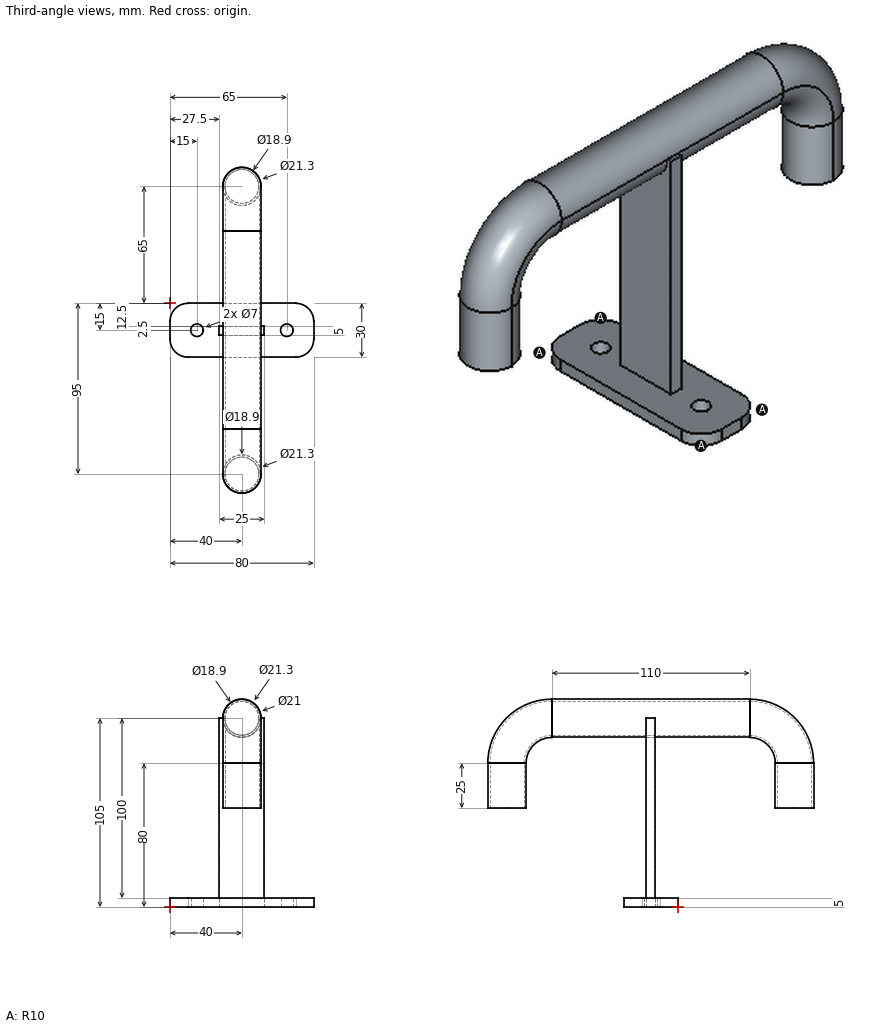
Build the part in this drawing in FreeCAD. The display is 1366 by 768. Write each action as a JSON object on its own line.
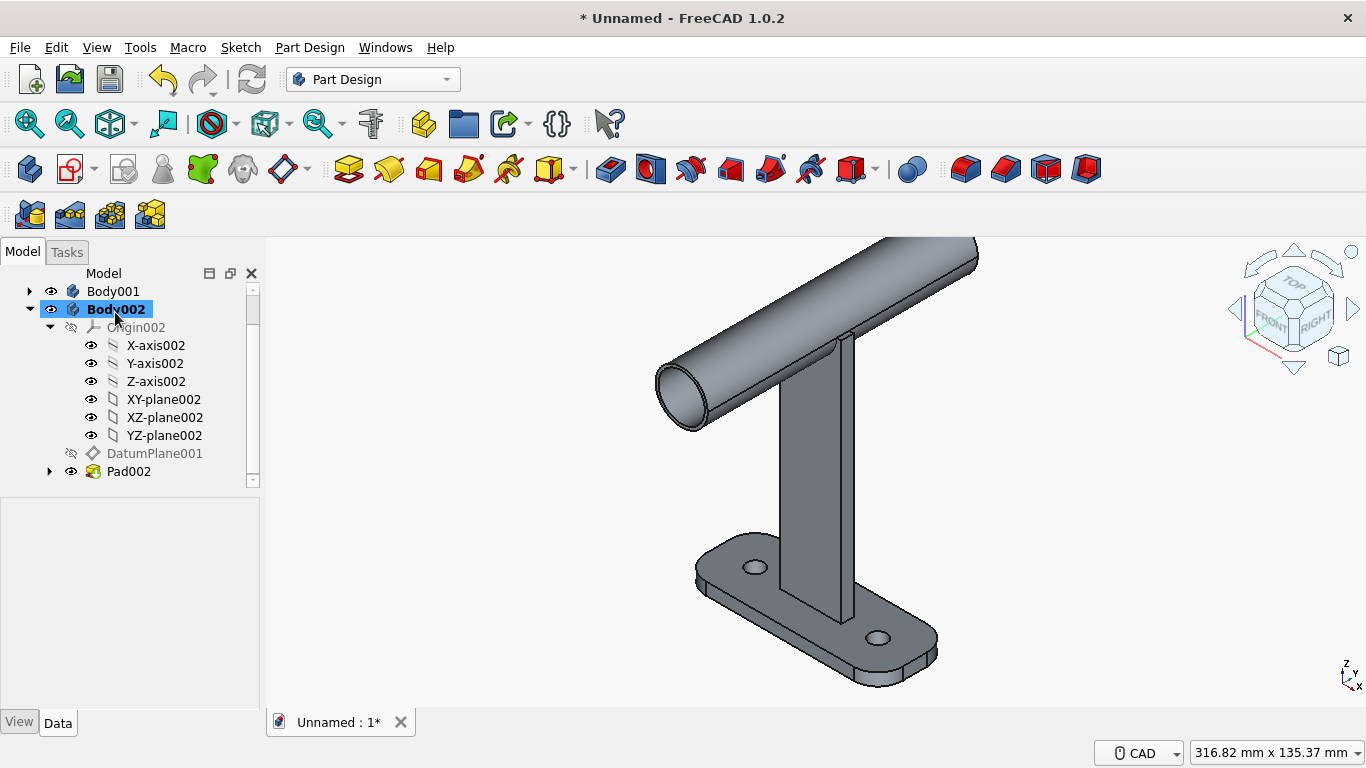
{"action": "left_click", "coordinate": [30, 124]}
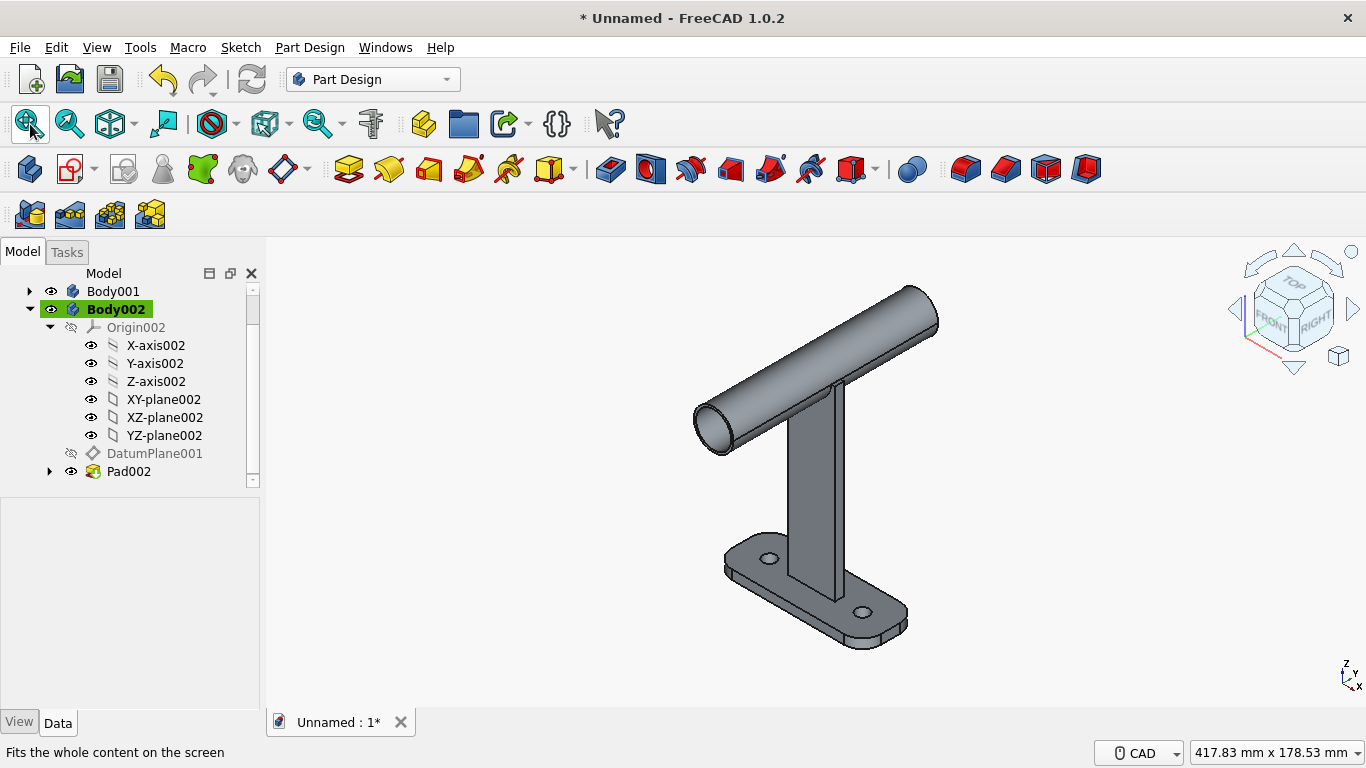
{"action": "left_click", "coordinate": [30, 170]}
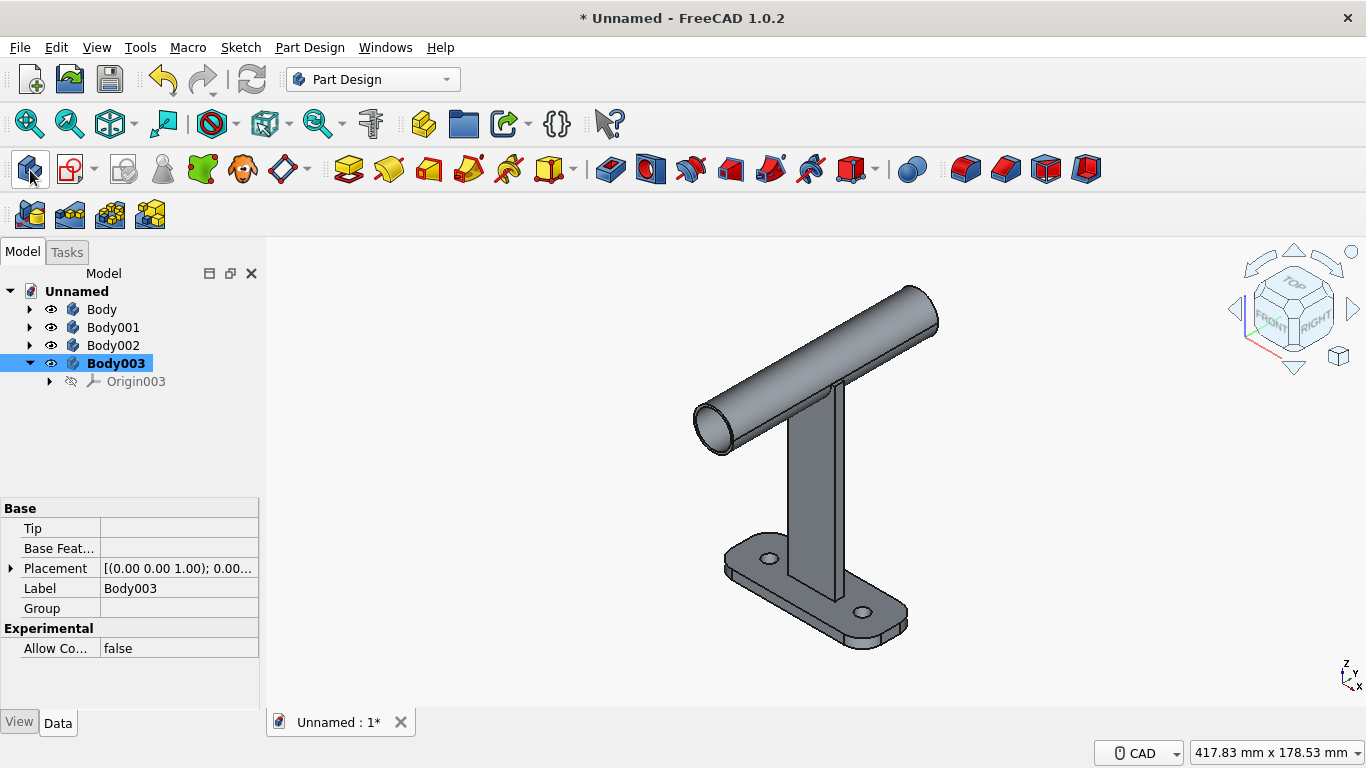
{"action": "left_click", "coordinate": [50, 381]}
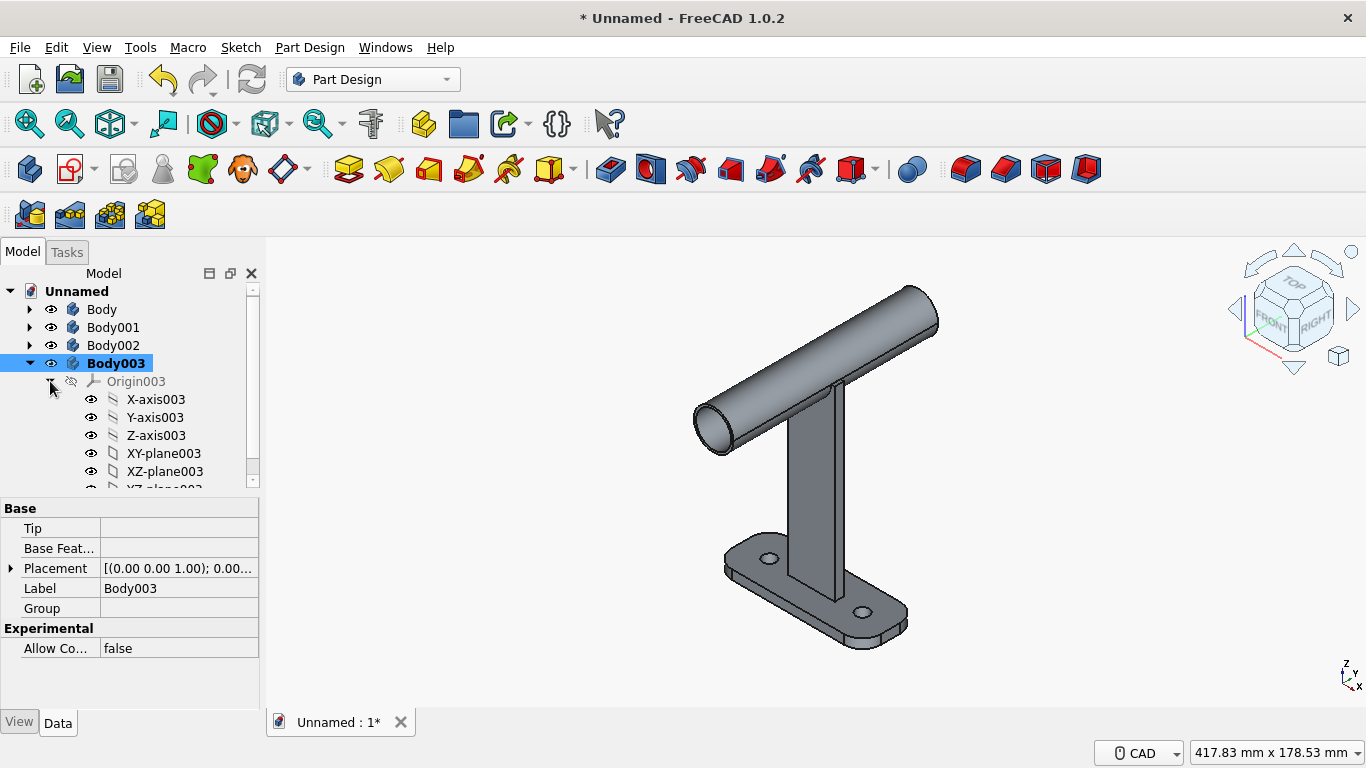
{"action": "left_click", "coordinate": [136, 471]}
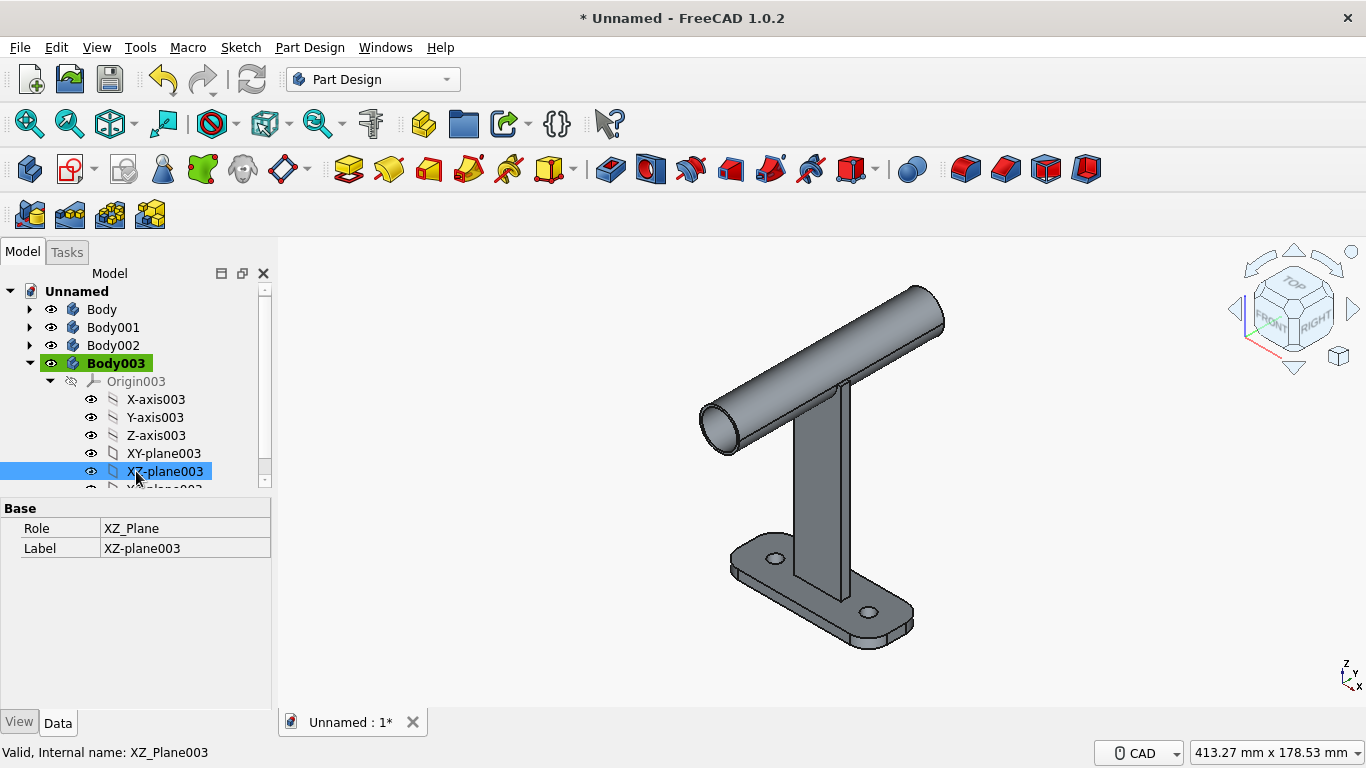
{"action": "left_click", "coordinate": [284, 170]}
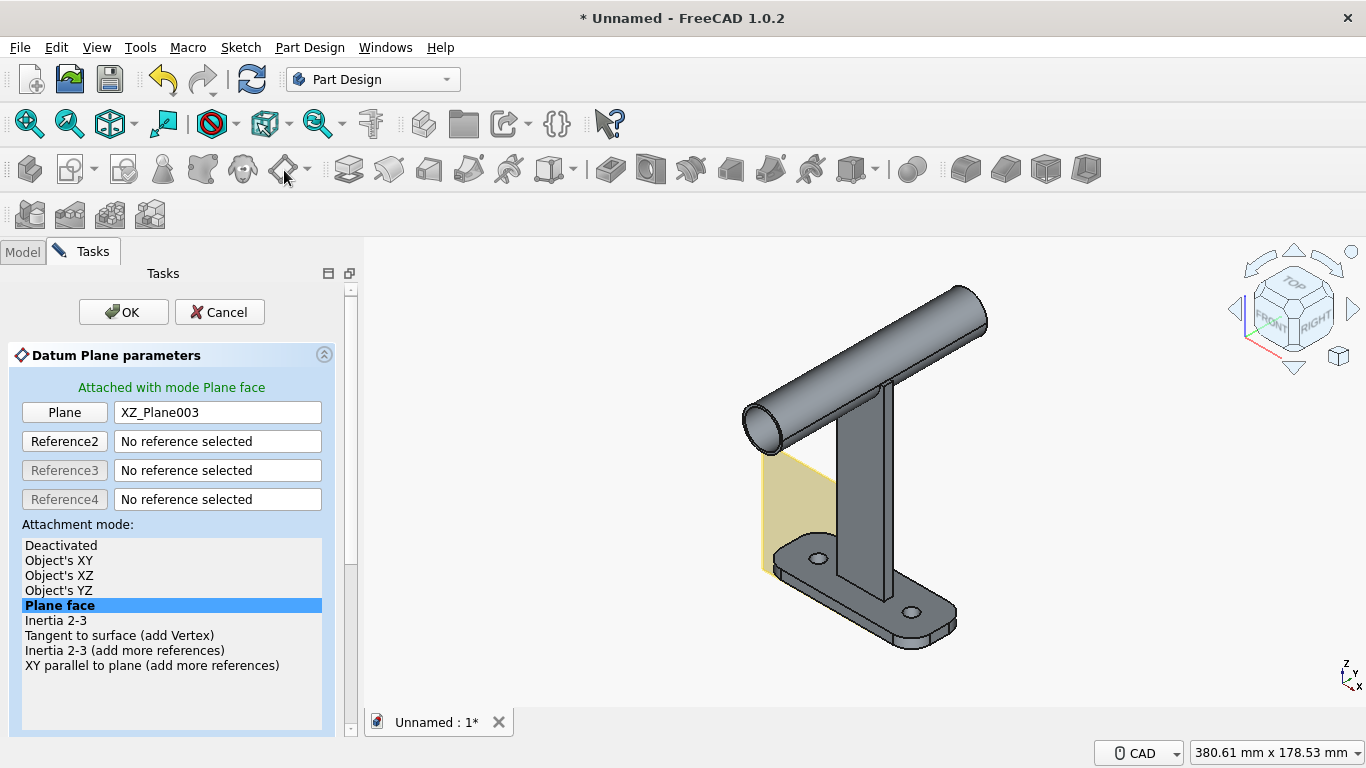
{"action": "scroll", "coordinate": [351, 510], "scroll_direction": "down", "scroll_amount": 3}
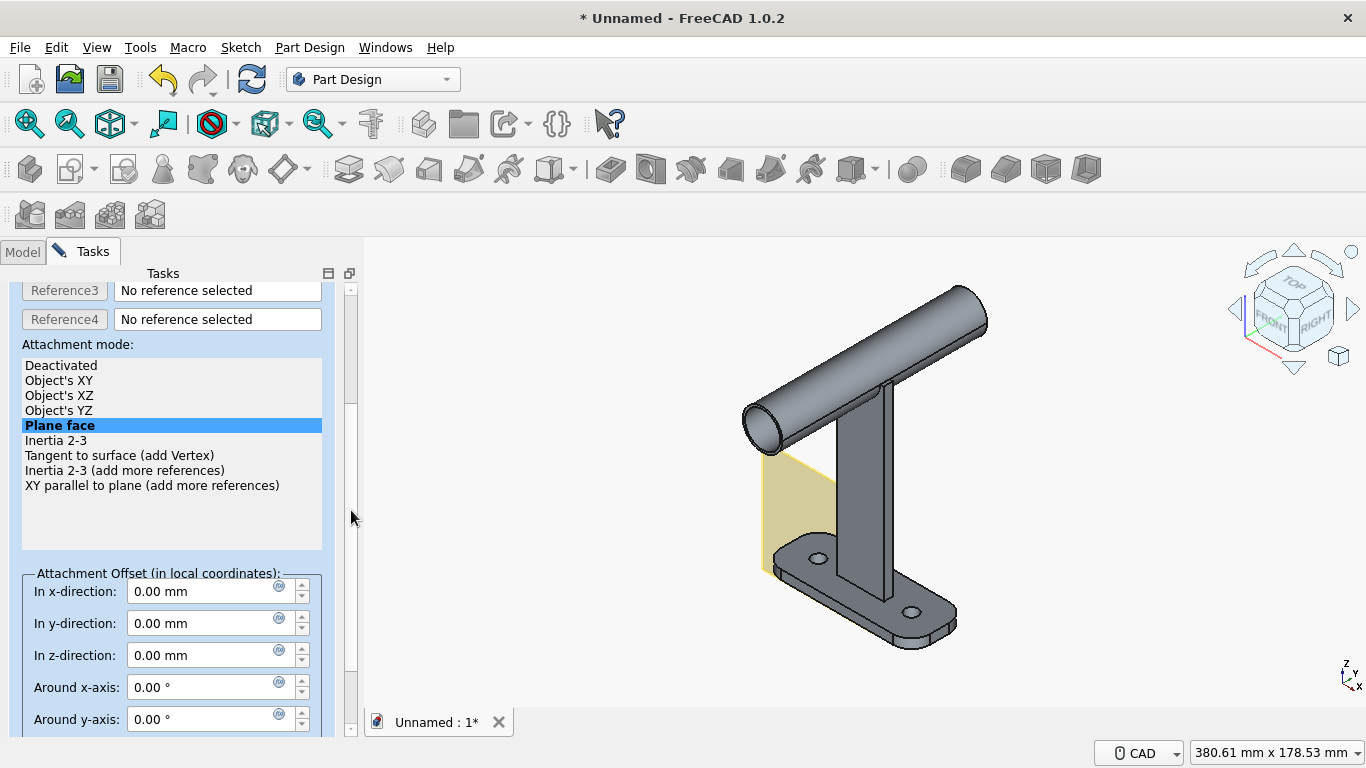
{"action": "triple_click", "coordinate": [210, 655]}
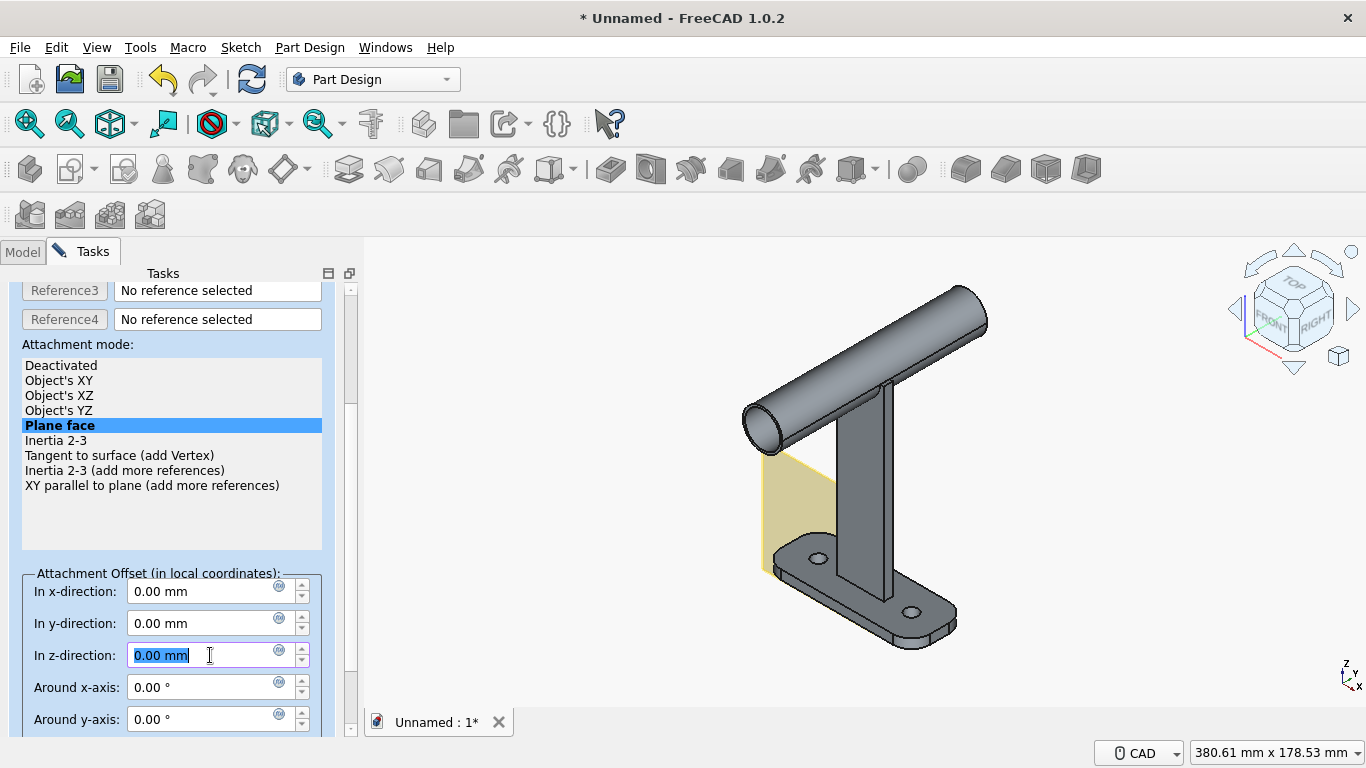
{"action": "type", "text": "-40"}
{"action": "key", "text": "Tab"}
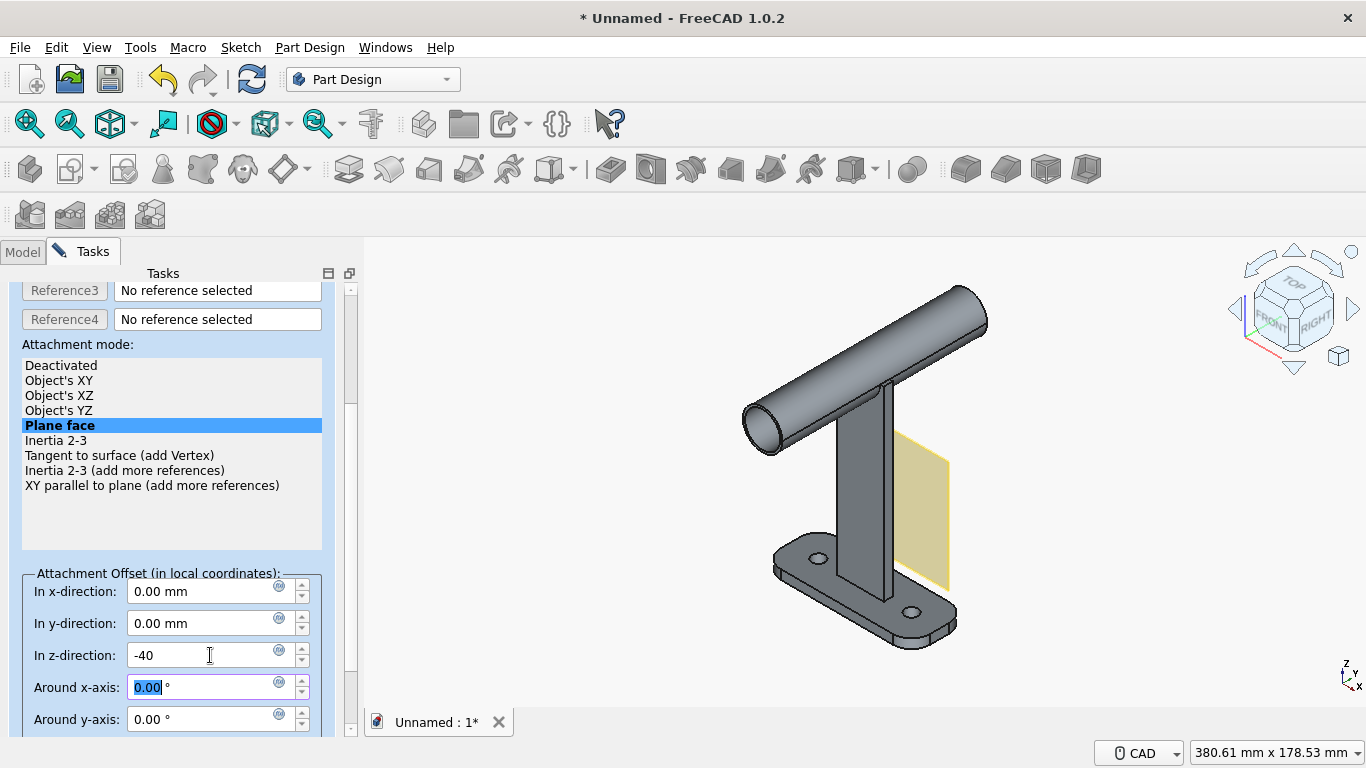
{"action": "scroll", "coordinate": [351, 510], "scroll_direction": "up", "scroll_amount": 4}